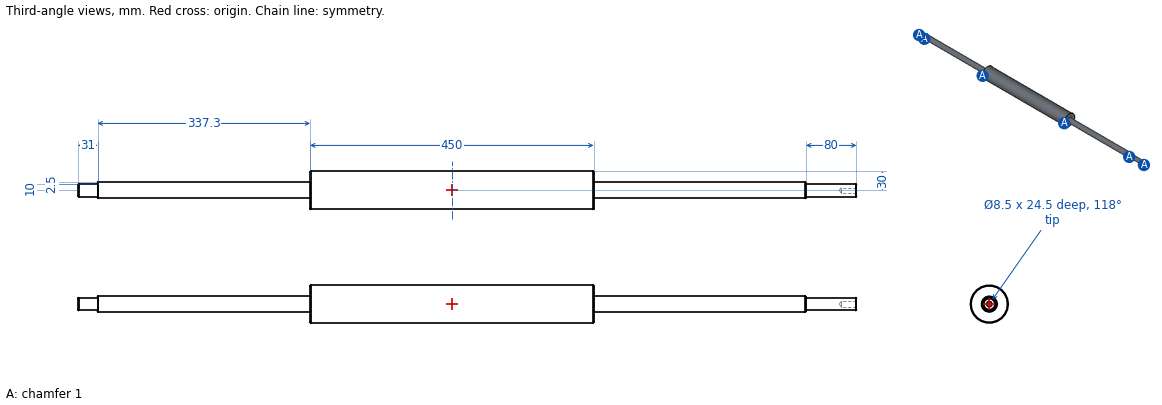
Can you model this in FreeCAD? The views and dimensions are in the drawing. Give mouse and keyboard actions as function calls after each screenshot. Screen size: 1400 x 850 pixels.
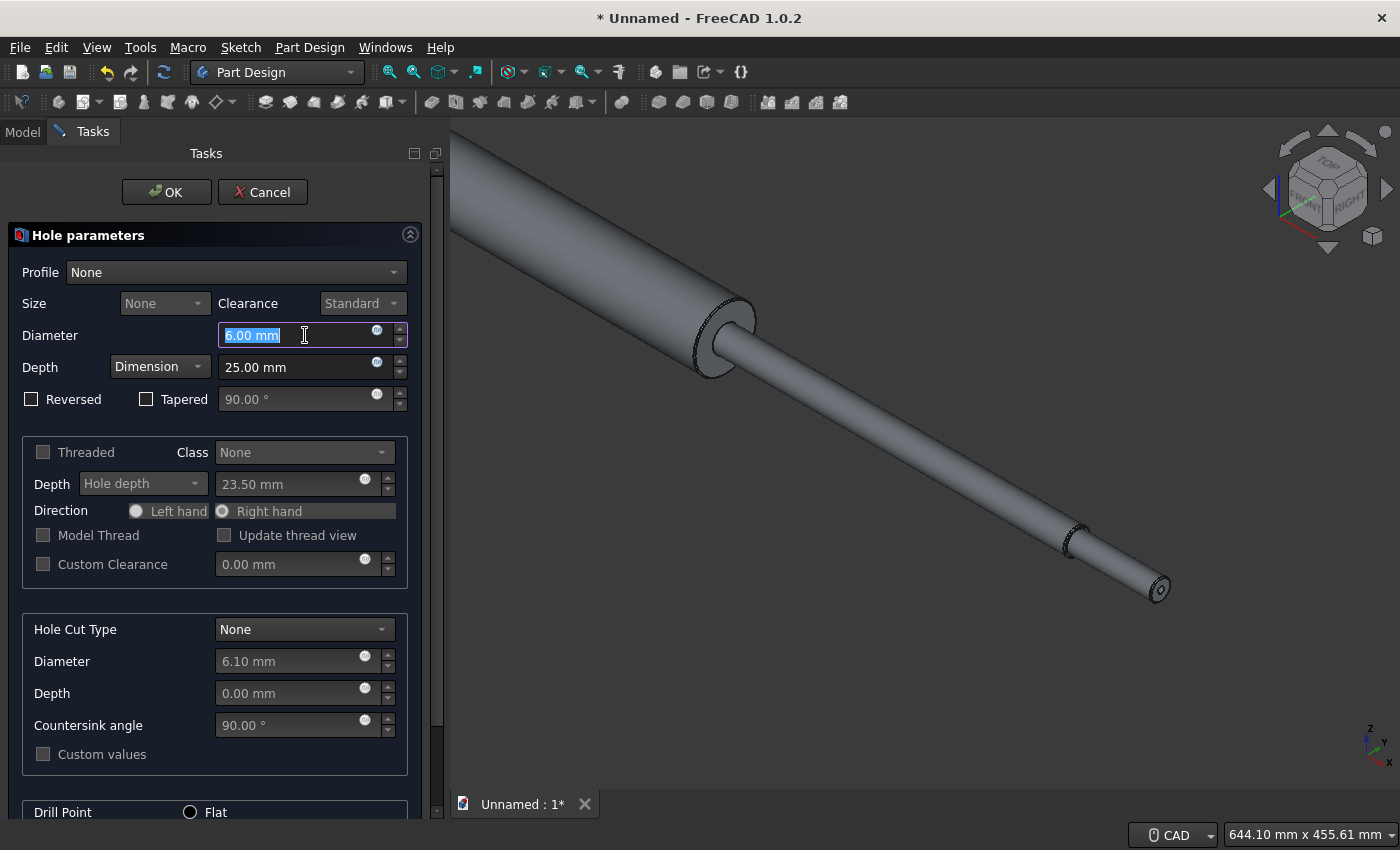
text(8.5)
key(Tab)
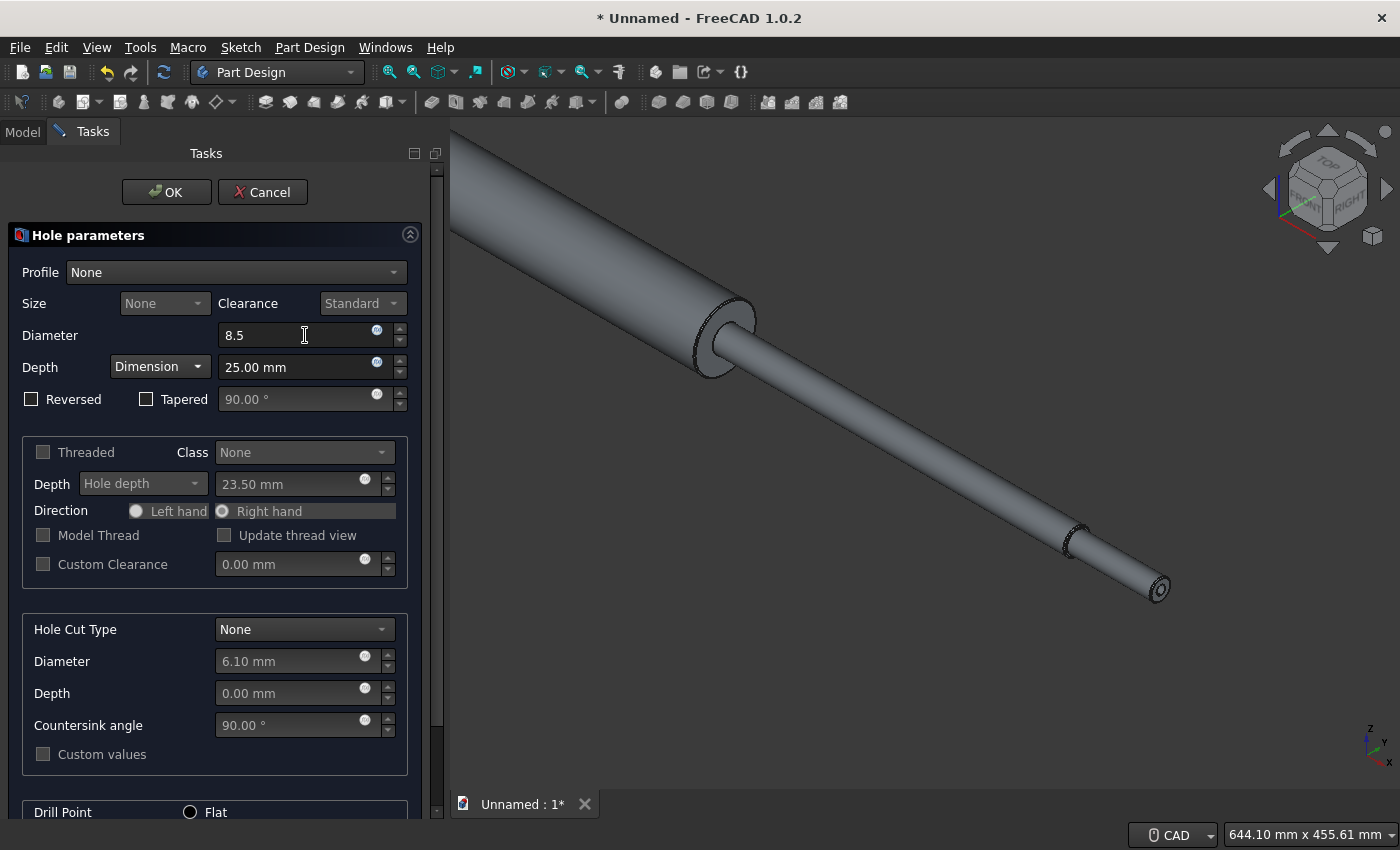
triple_click(305, 367)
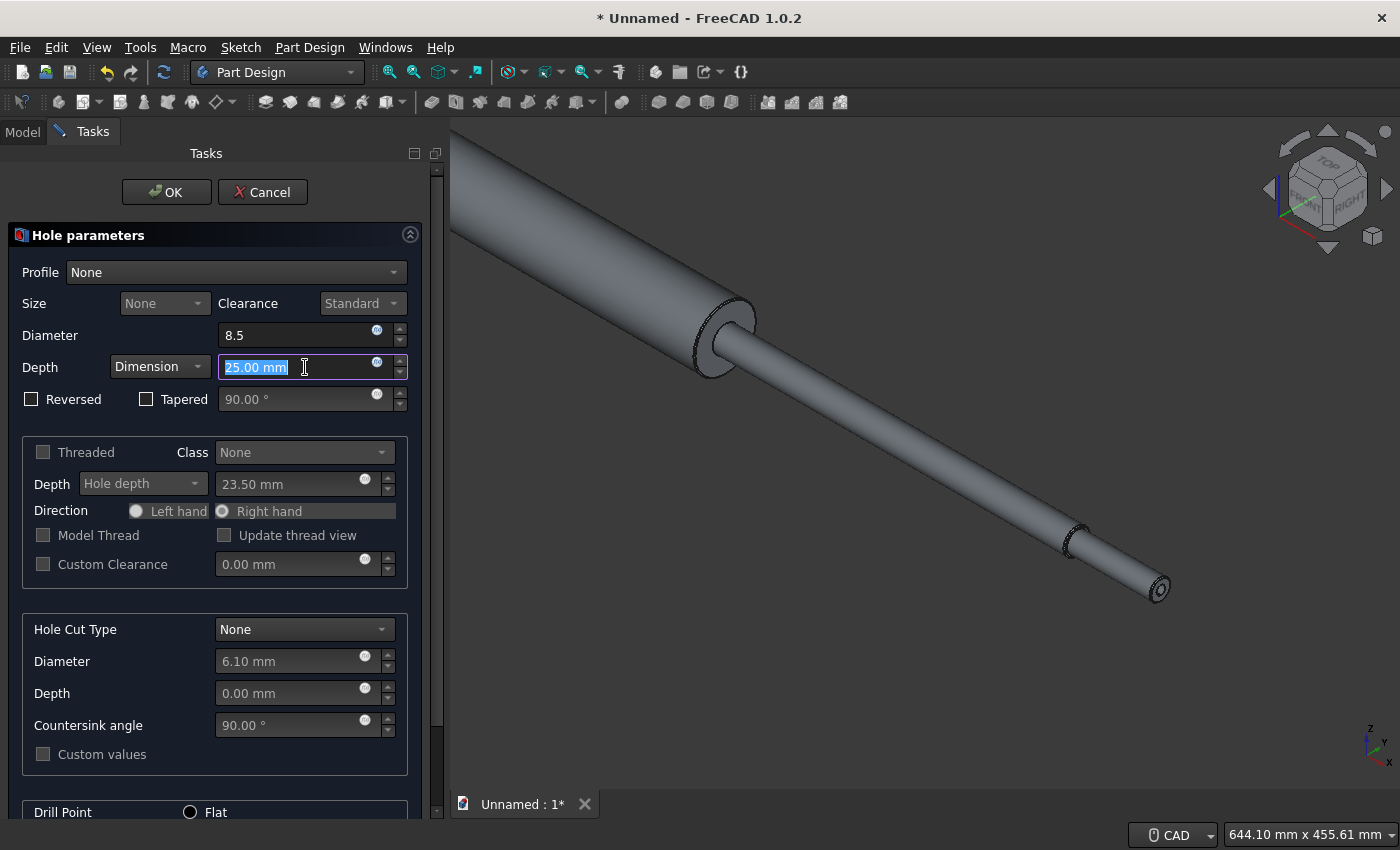
text(24.5)
key(Tab)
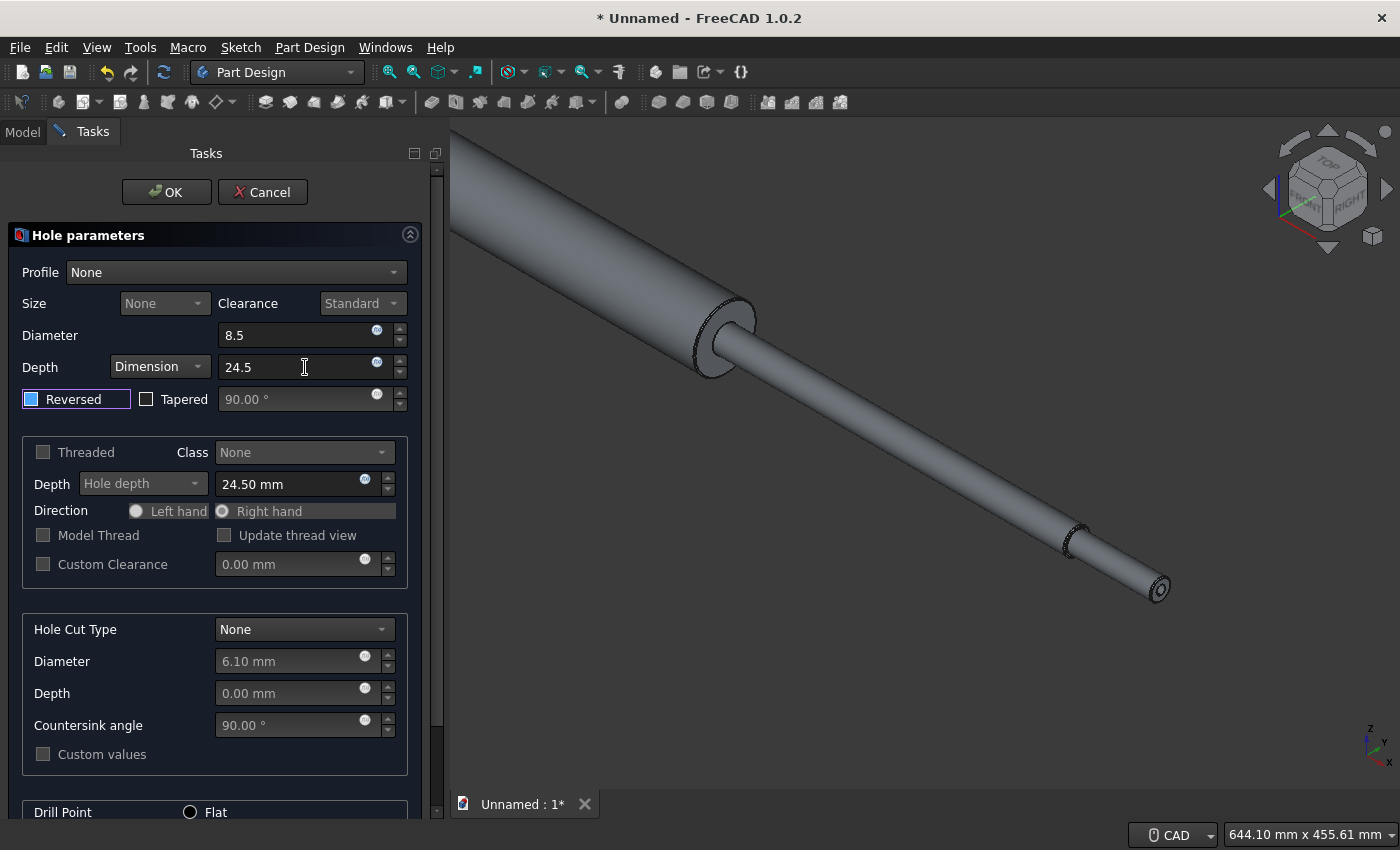
click(167, 192)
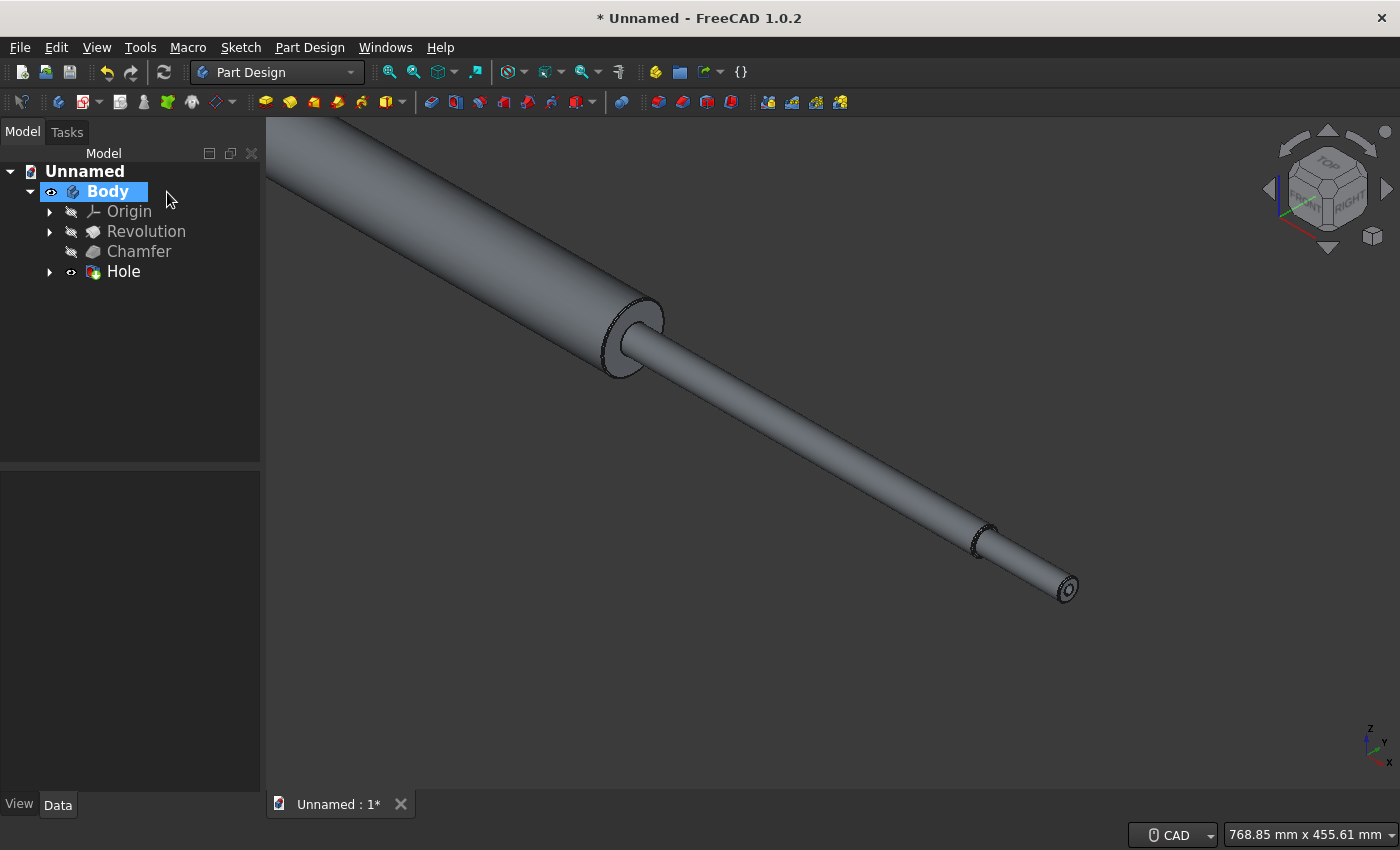
key(v)
key(f)